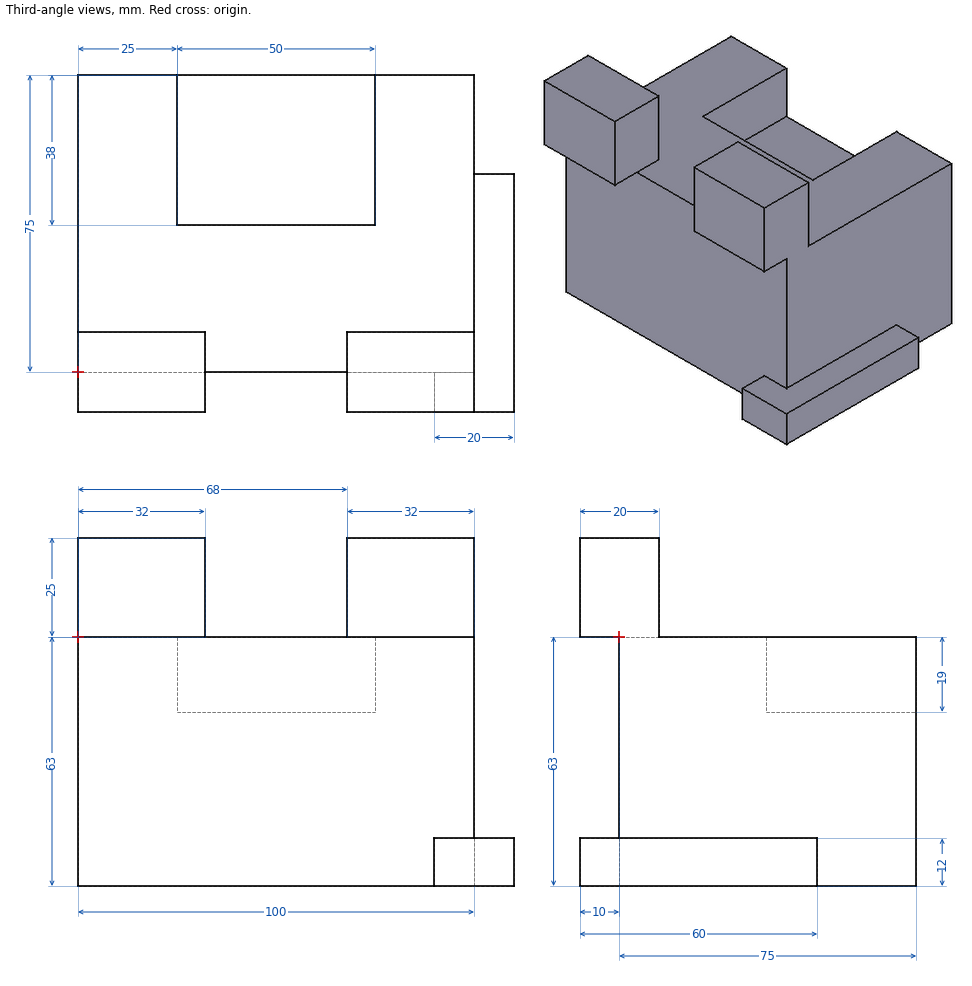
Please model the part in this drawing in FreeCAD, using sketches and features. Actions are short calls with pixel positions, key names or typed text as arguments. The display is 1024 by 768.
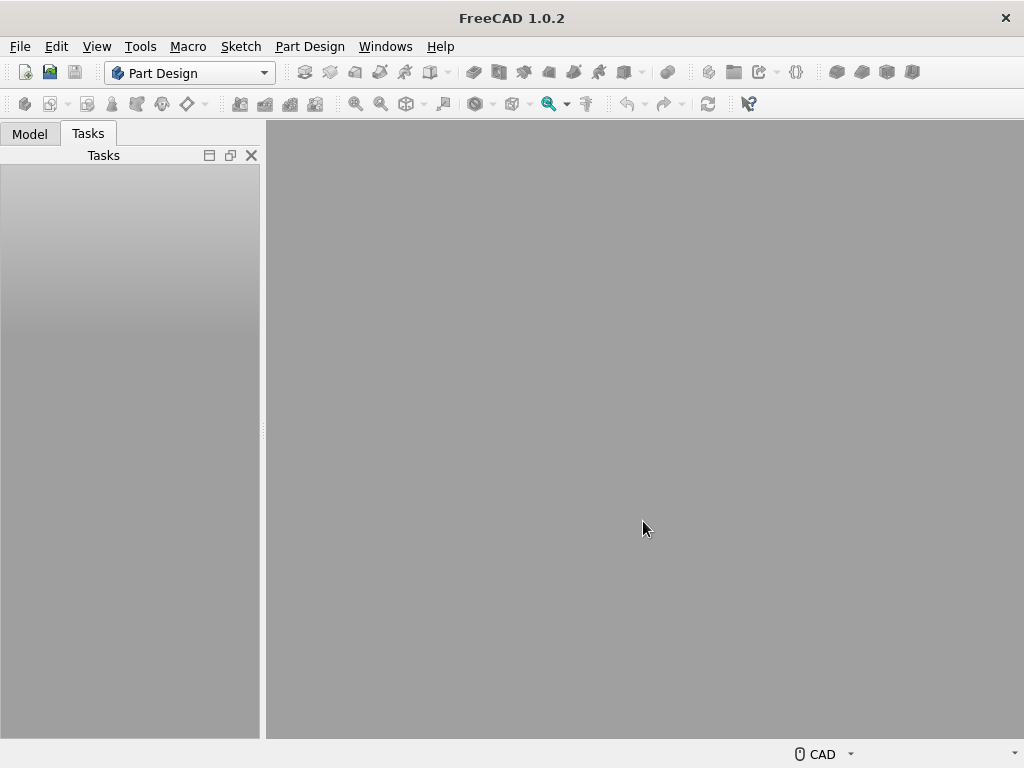
click(25, 72)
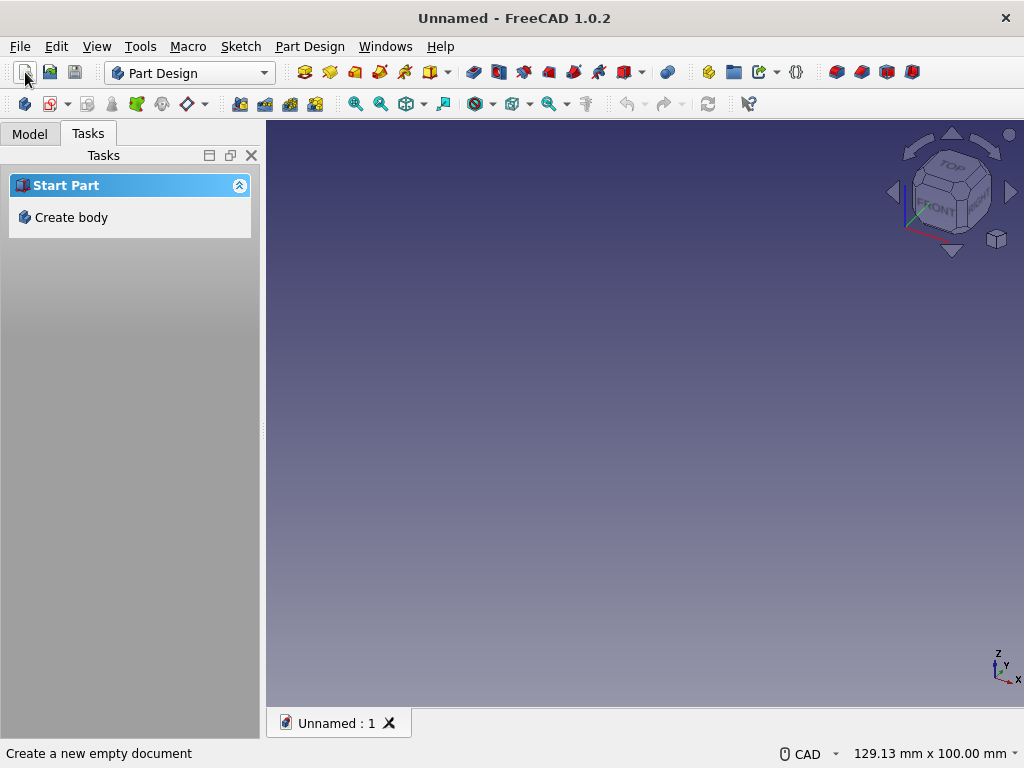
click(50, 104)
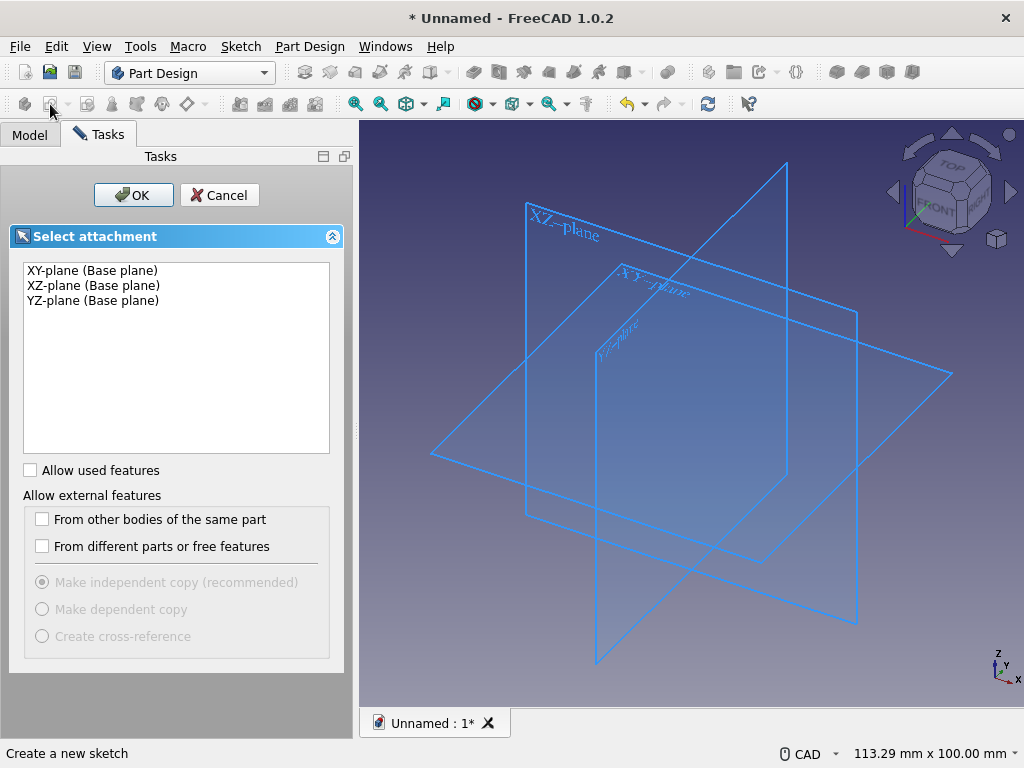
click(84, 286)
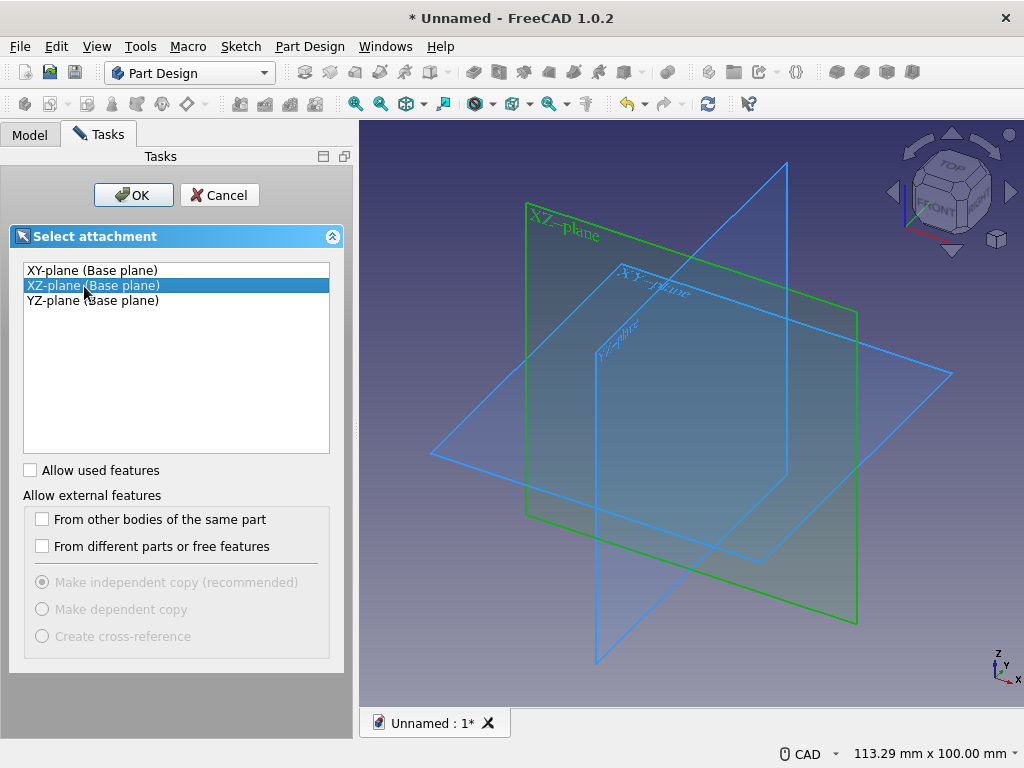
click(134, 195)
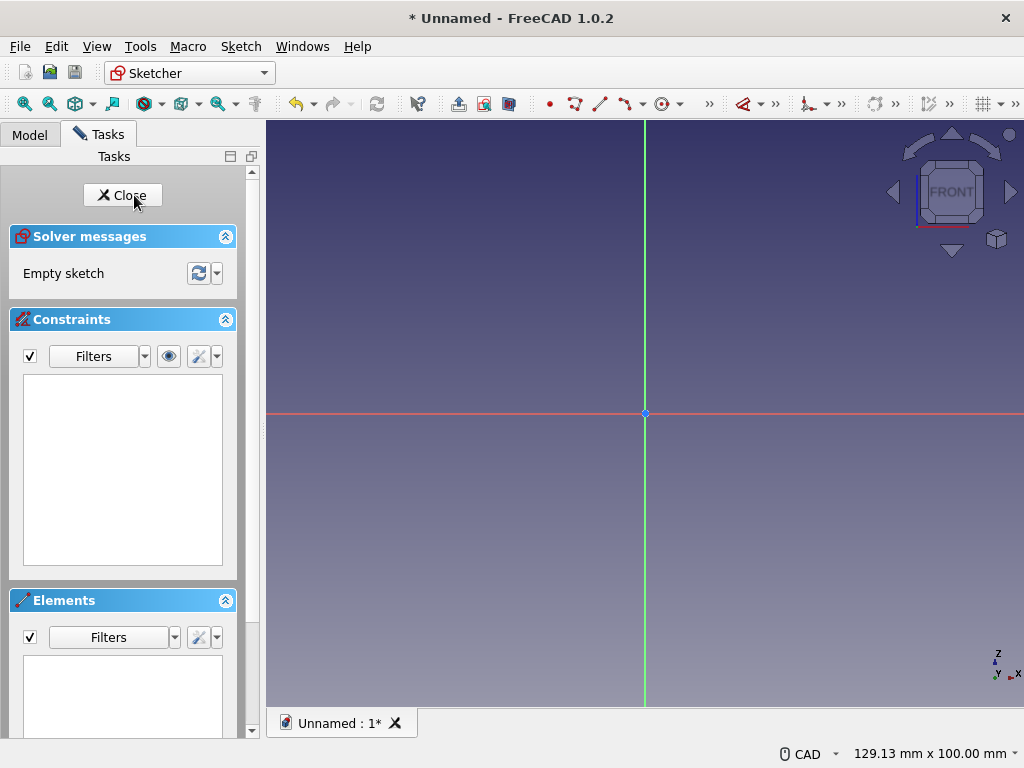
scroll(294, 189, down, 3)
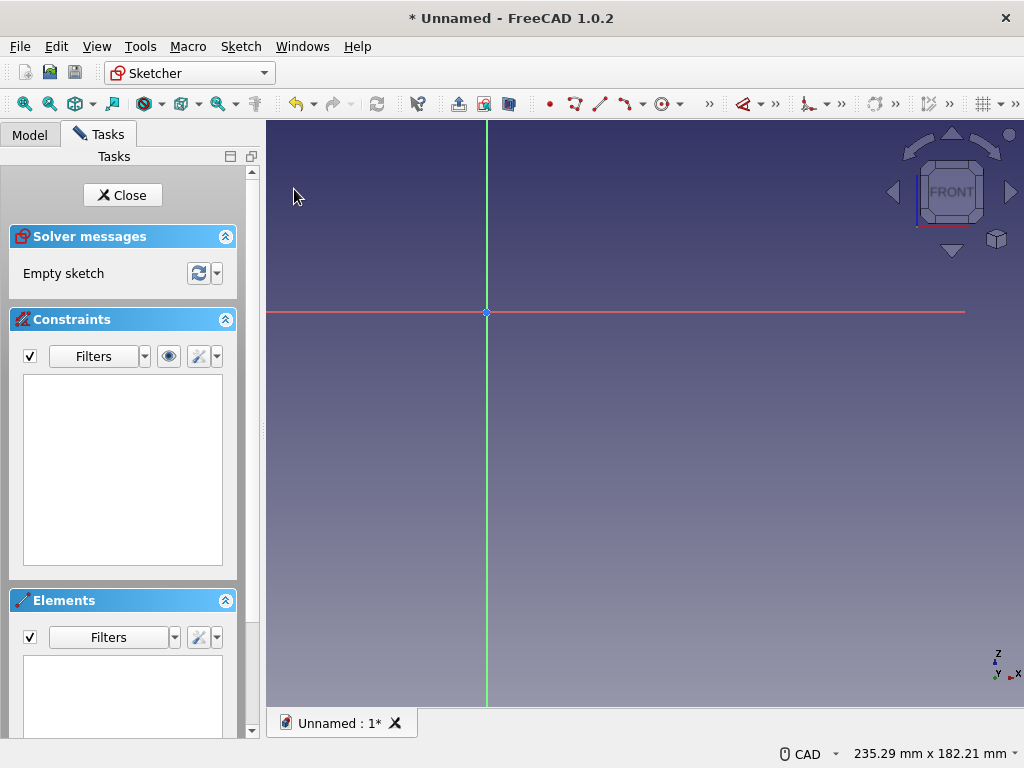
key(g)
key(r)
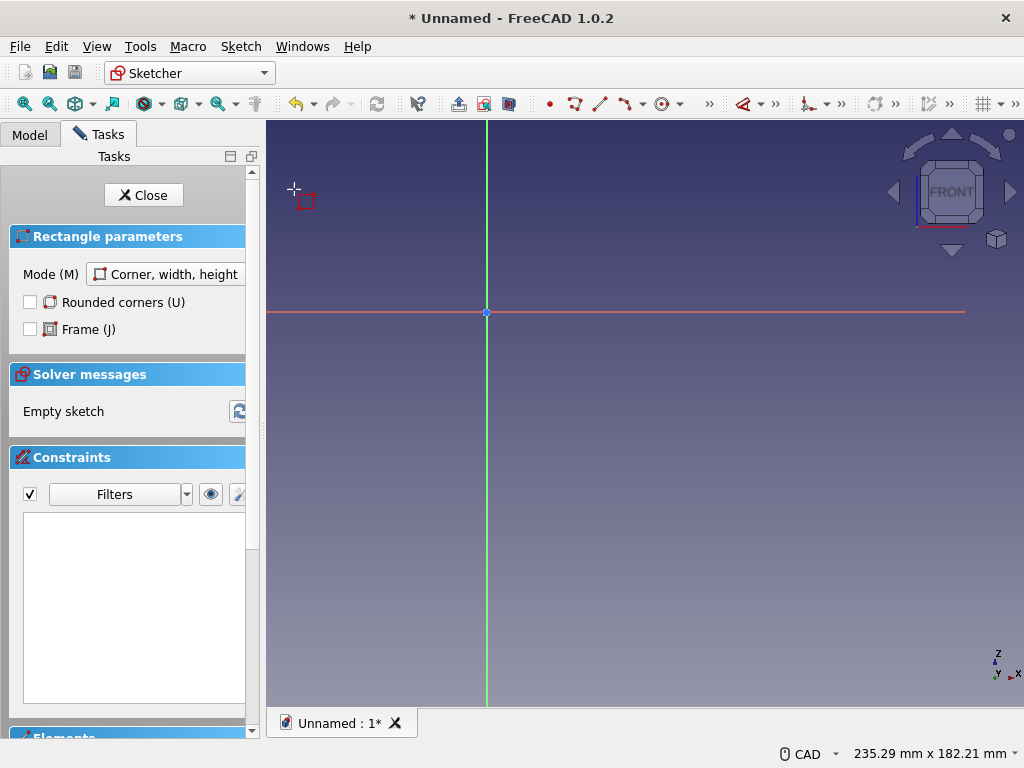
click(487, 312)
click(809, 515)
key(Escape)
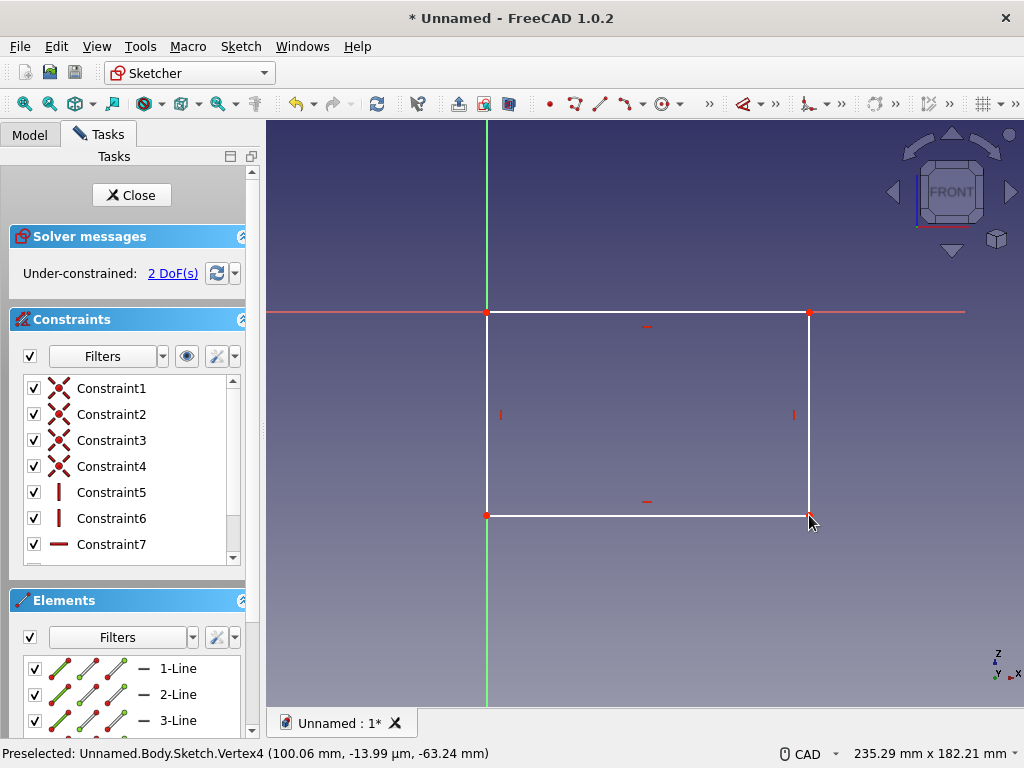
click(742, 104)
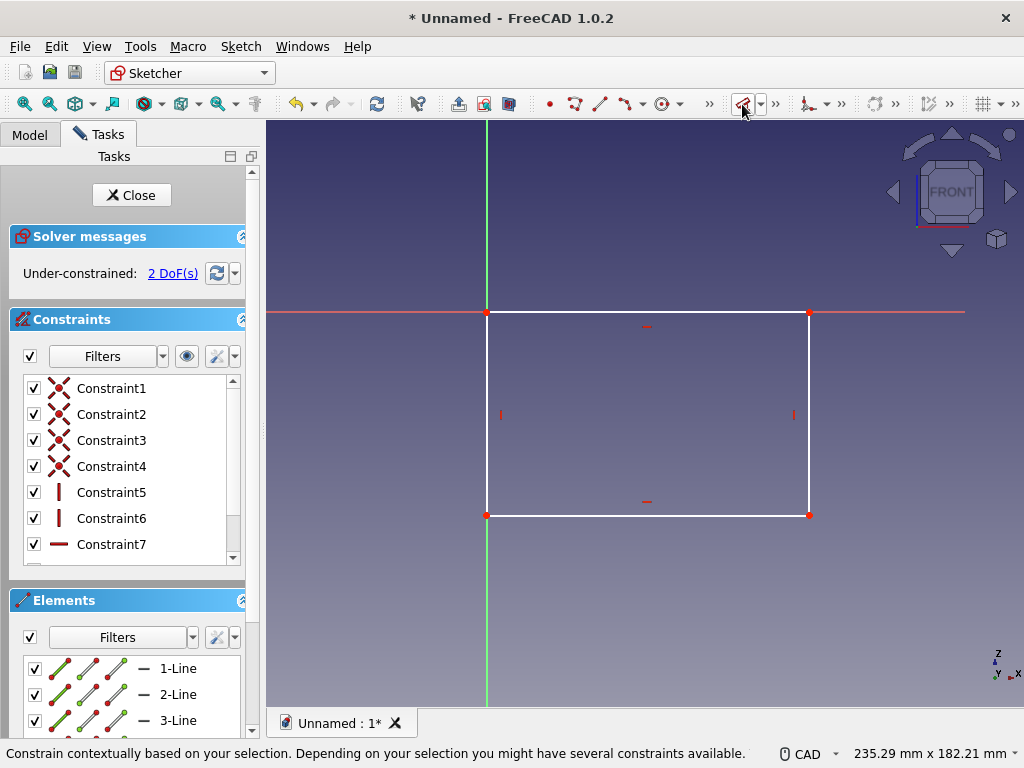
click(487, 373)
click(453, 414)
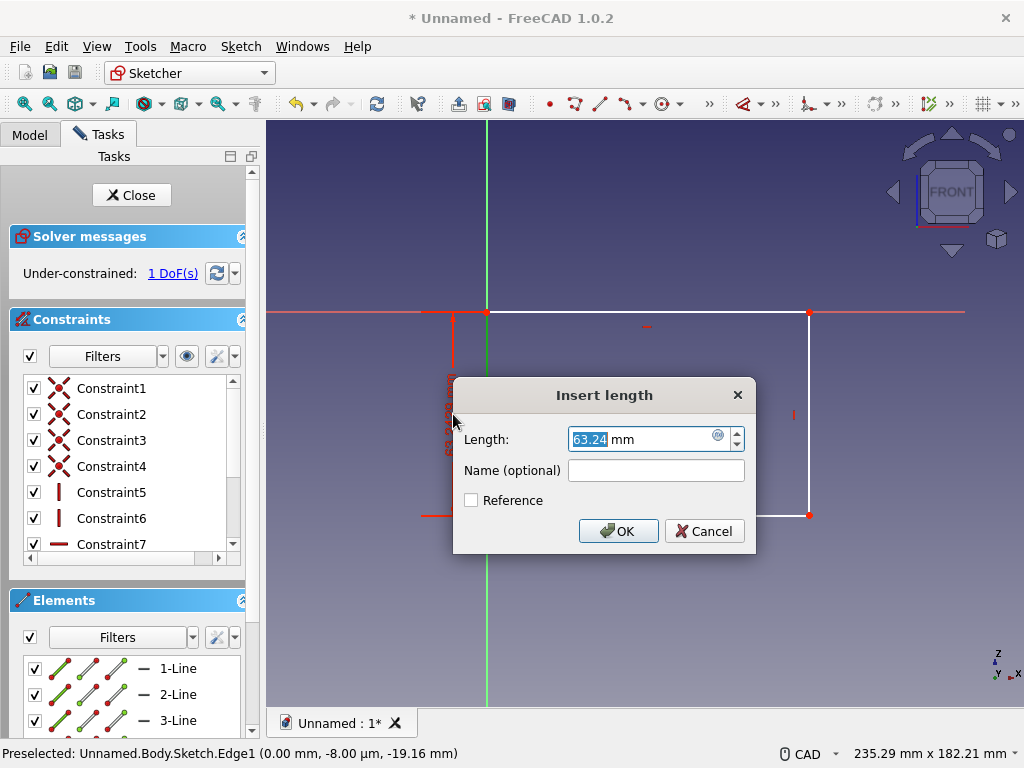
text(63)
key(Return)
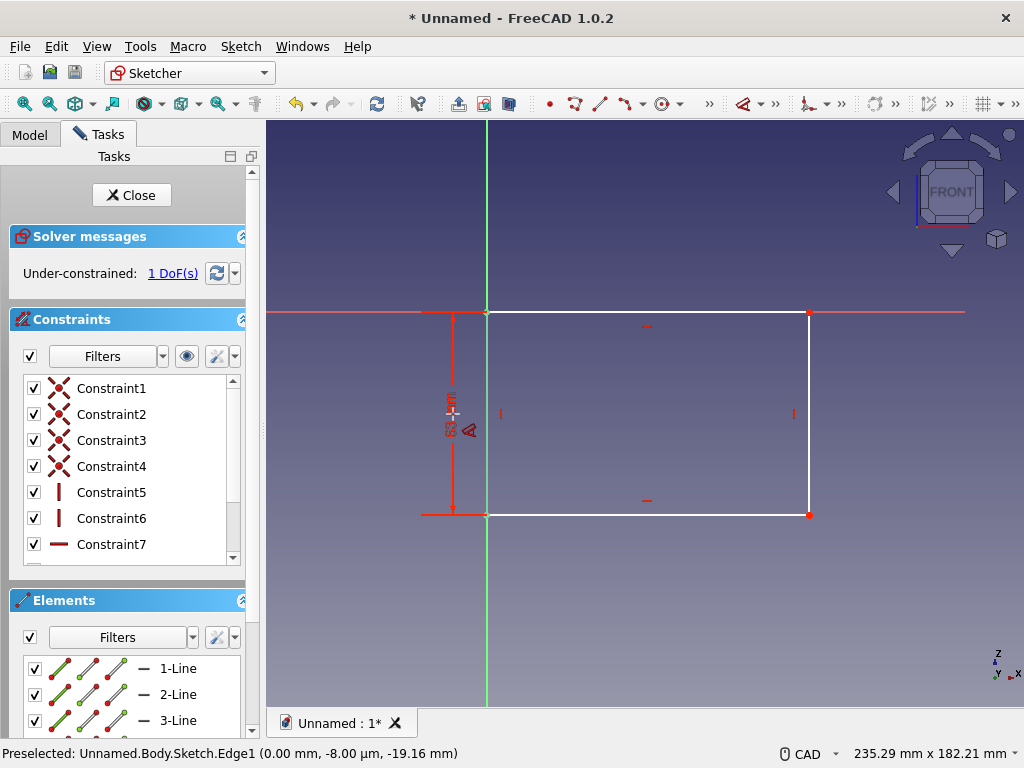
click(583, 515)
click(648, 549)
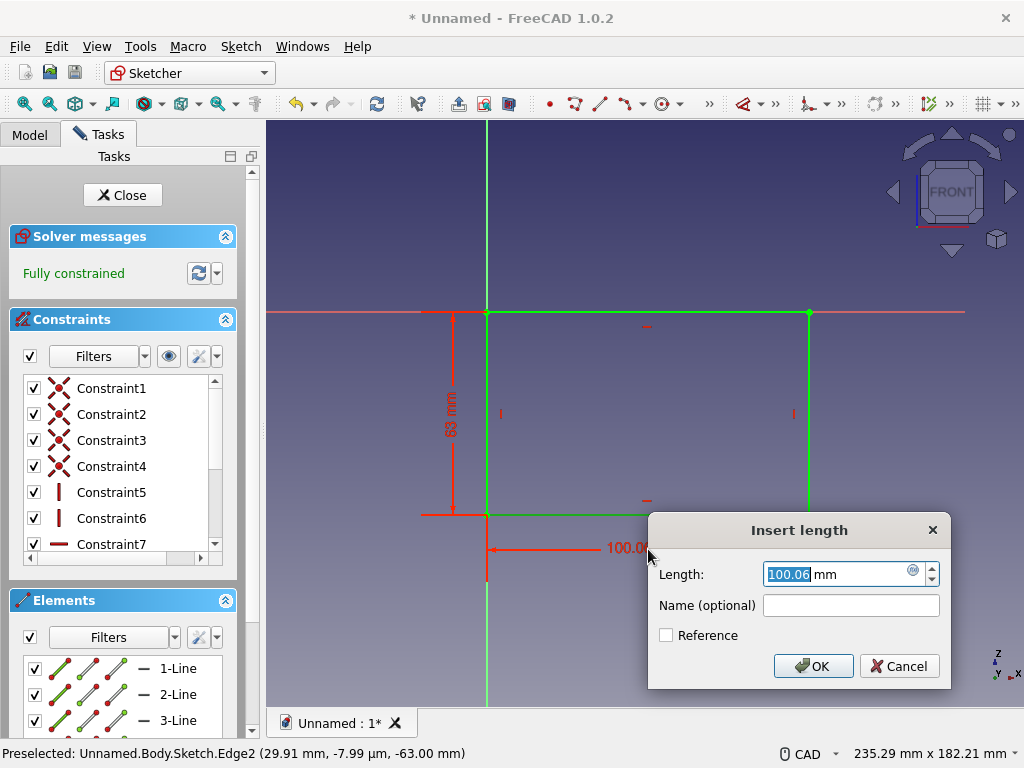
text(100)
key(Return)
key(Escape)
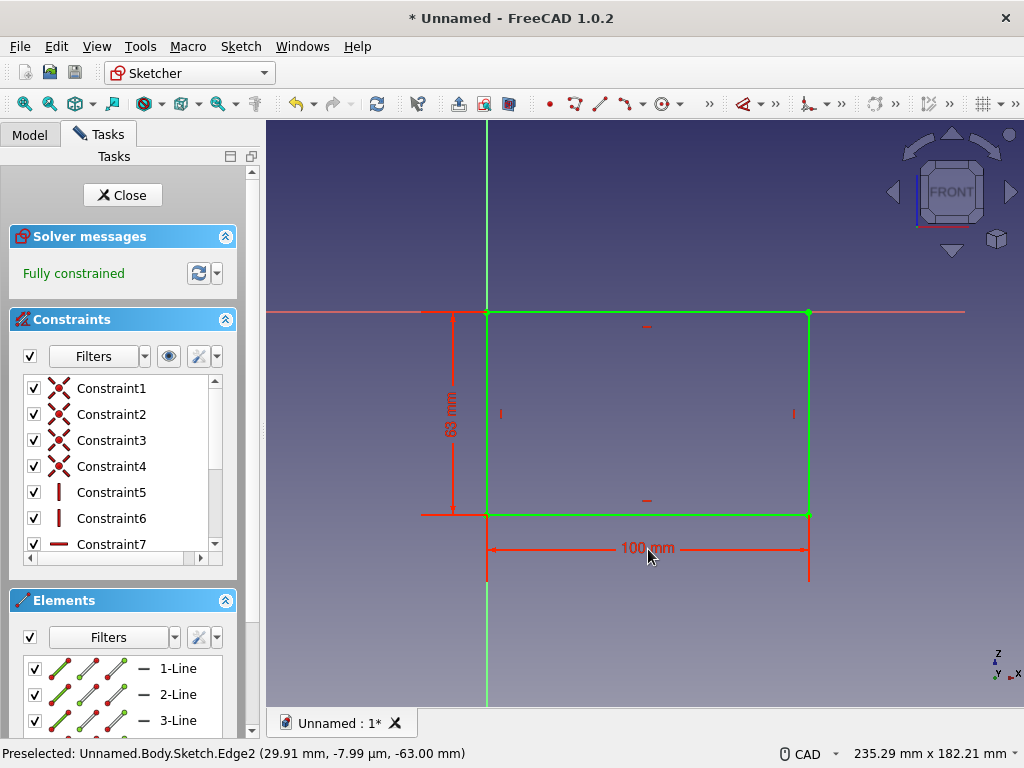
click(123, 195)